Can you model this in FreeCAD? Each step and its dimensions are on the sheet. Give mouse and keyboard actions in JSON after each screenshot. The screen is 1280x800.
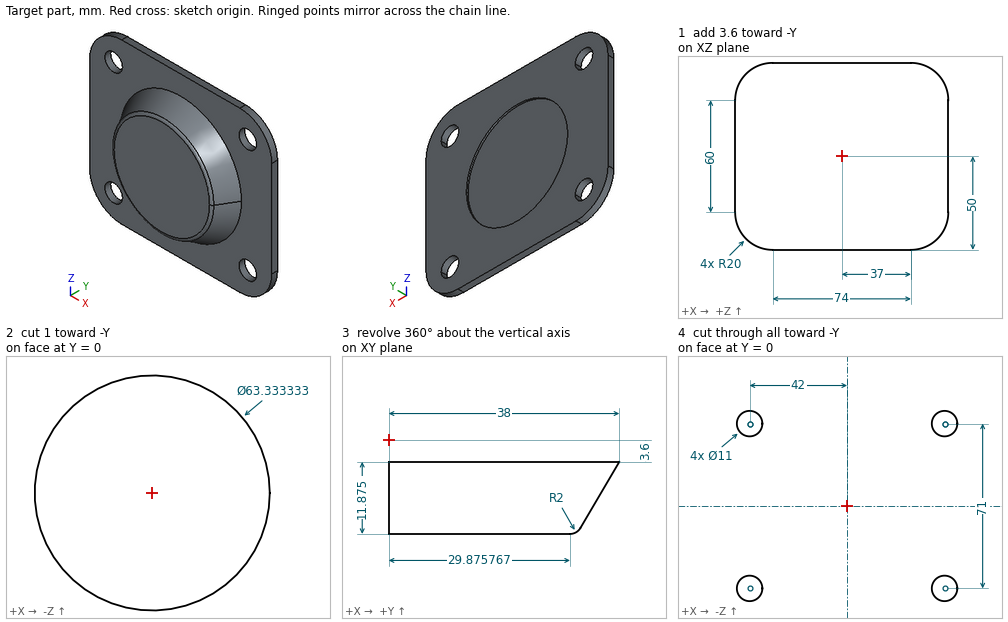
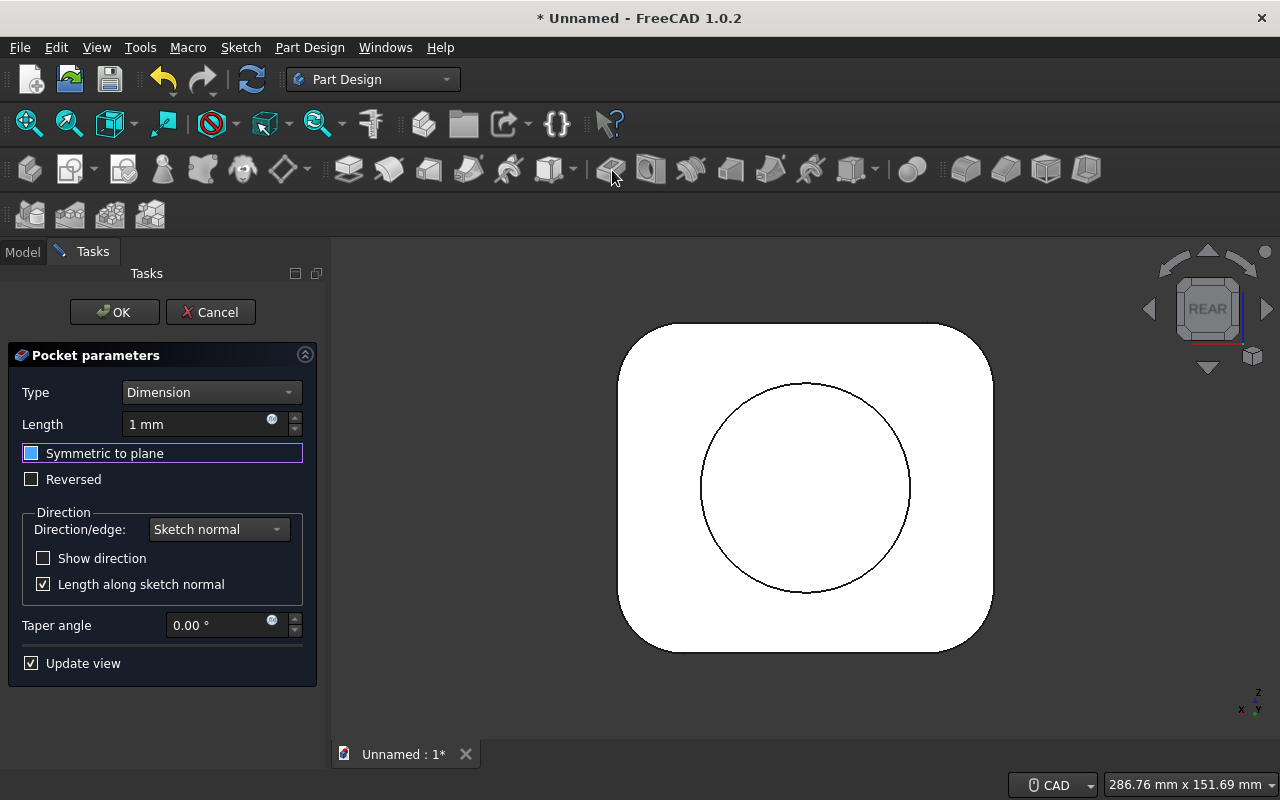
{"action": "left_click", "coordinate": [115, 312]}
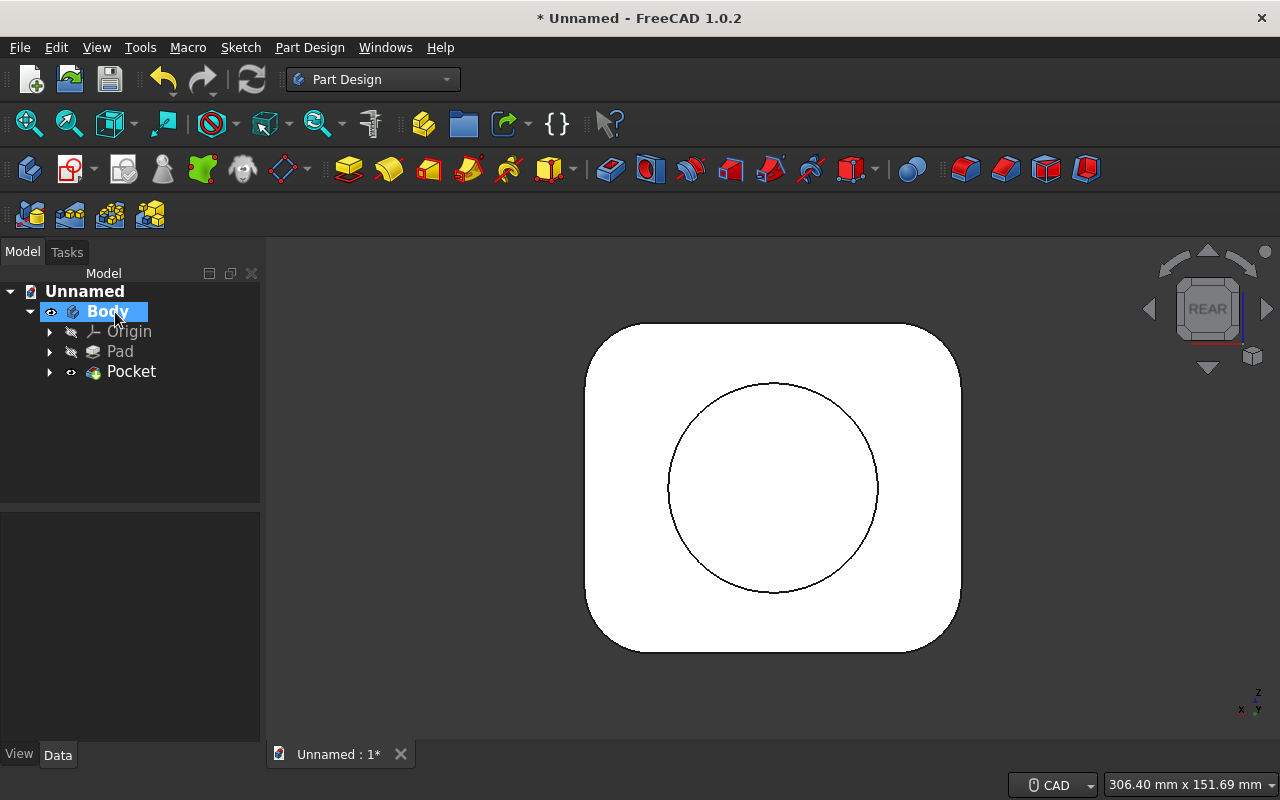
{"action": "left_click", "coordinate": [70, 170]}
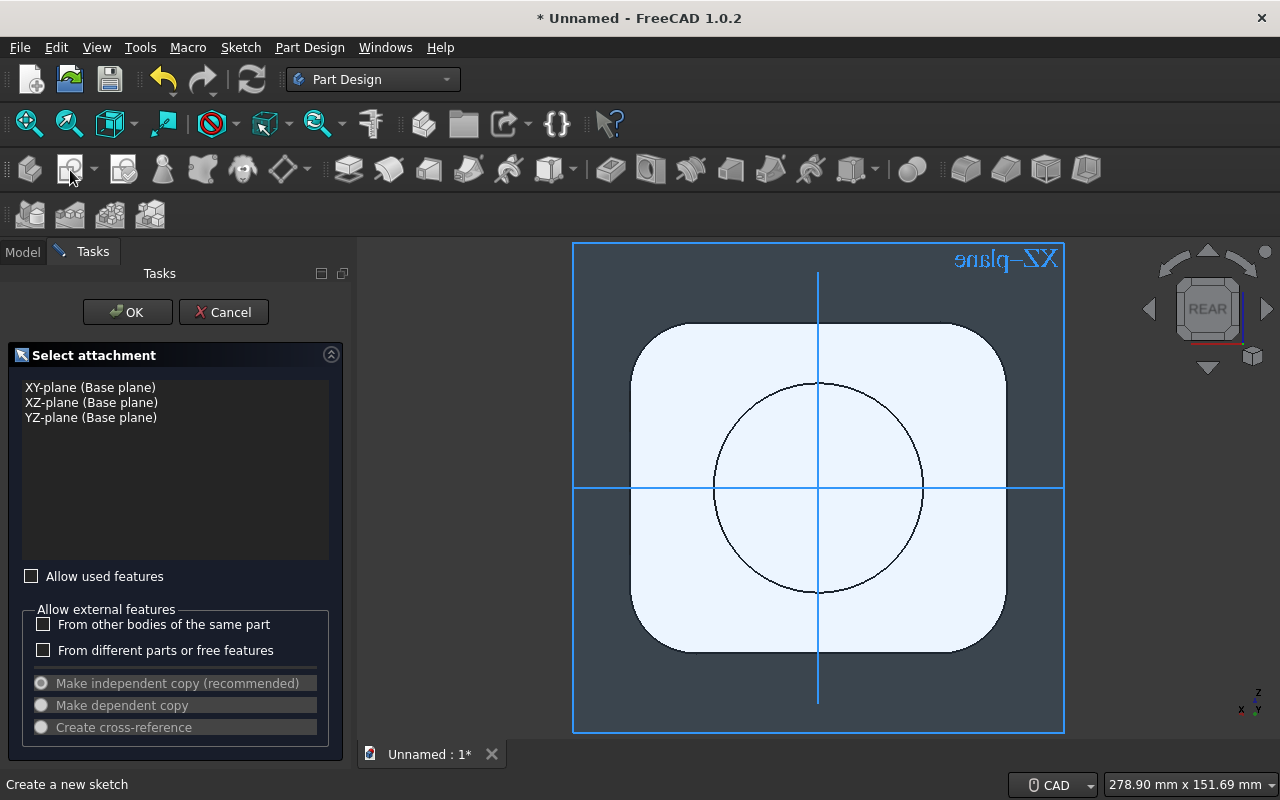
{"action": "left_click", "coordinate": [82, 388]}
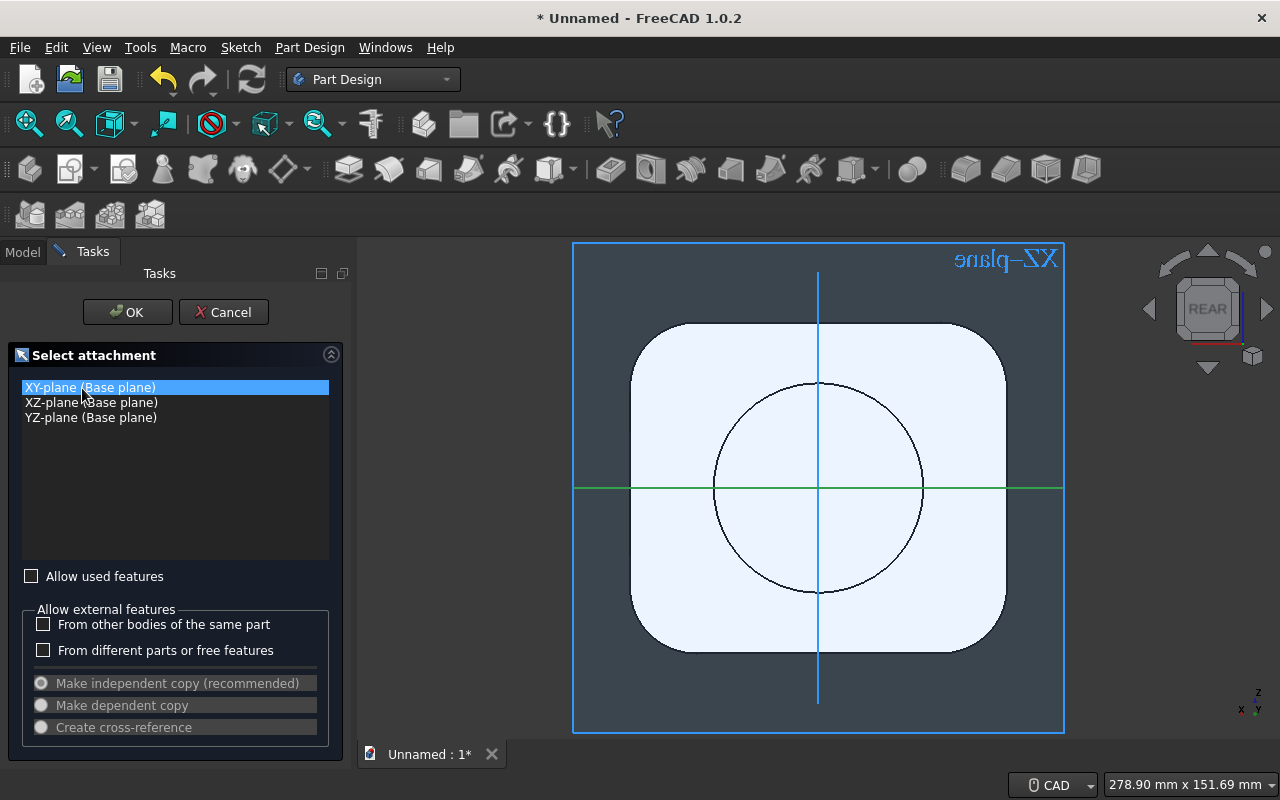
{"action": "left_click", "coordinate": [128, 312]}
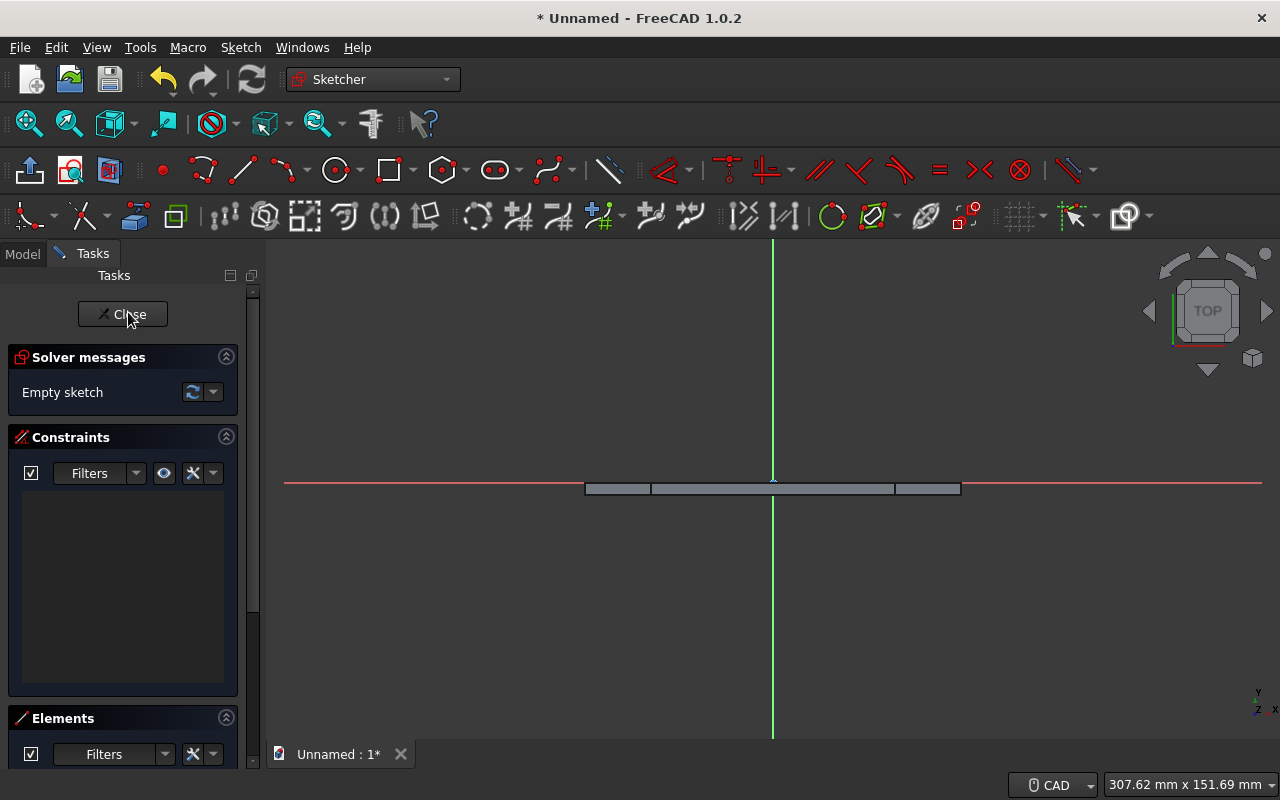
{"action": "left_click", "coordinate": [110, 170]}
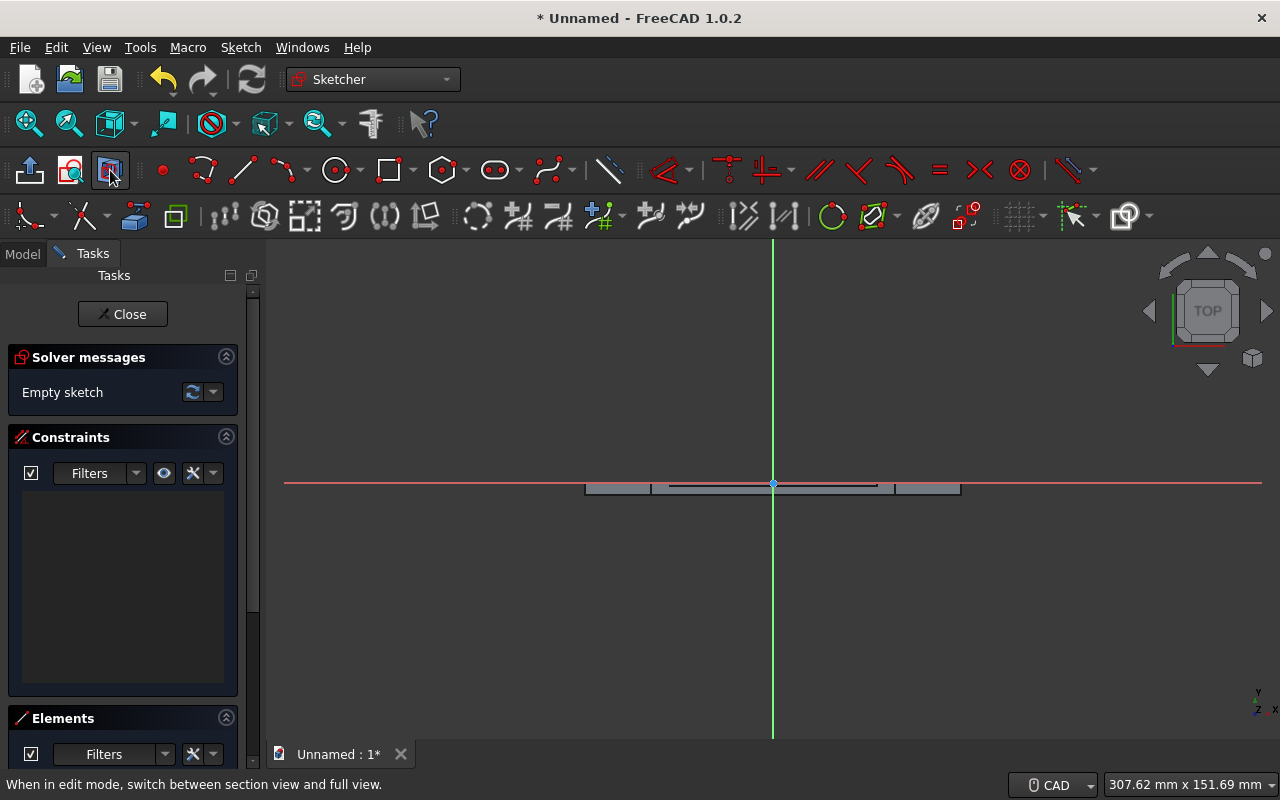
{"action": "scroll", "coordinate": [869, 514], "scroll_direction": "up", "scroll_amount": 8}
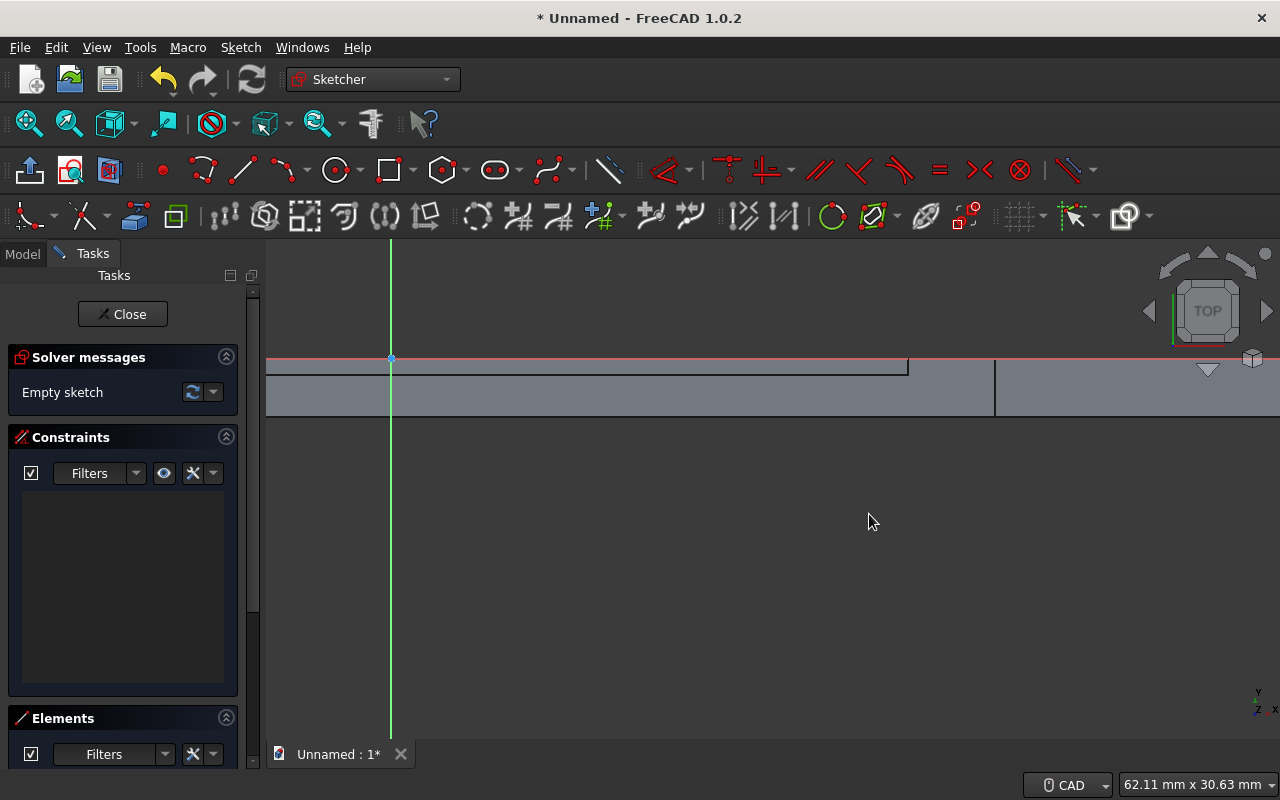
{"action": "left_click", "coordinate": [204, 170]}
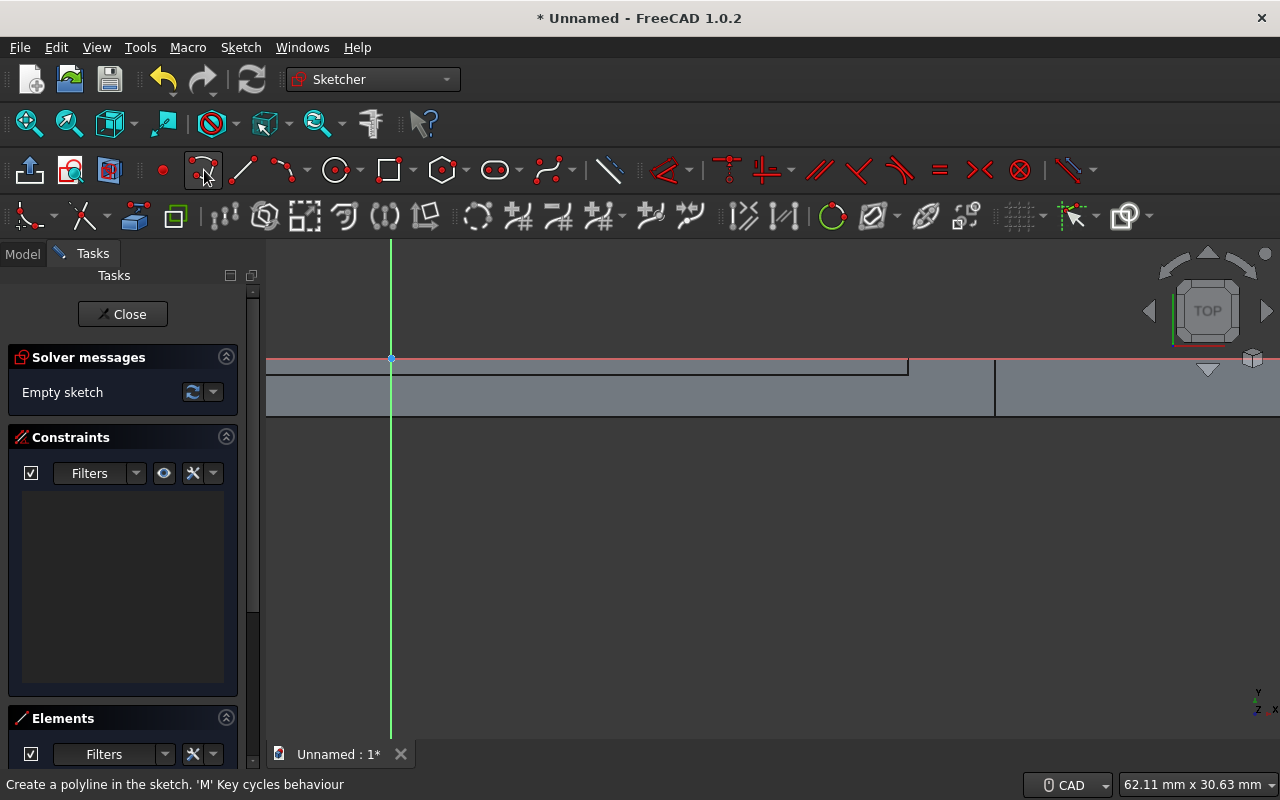
{"action": "left_click", "coordinate": [907, 595]}
{"action": "left_click", "coordinate": [1012, 417]}
{"action": "left_click", "coordinate": [391, 417]}
{"action": "left_click", "coordinate": [400, 611]}
{"action": "left_click", "coordinate": [879, 611]}
{"action": "right_click", "coordinate": [879, 611]}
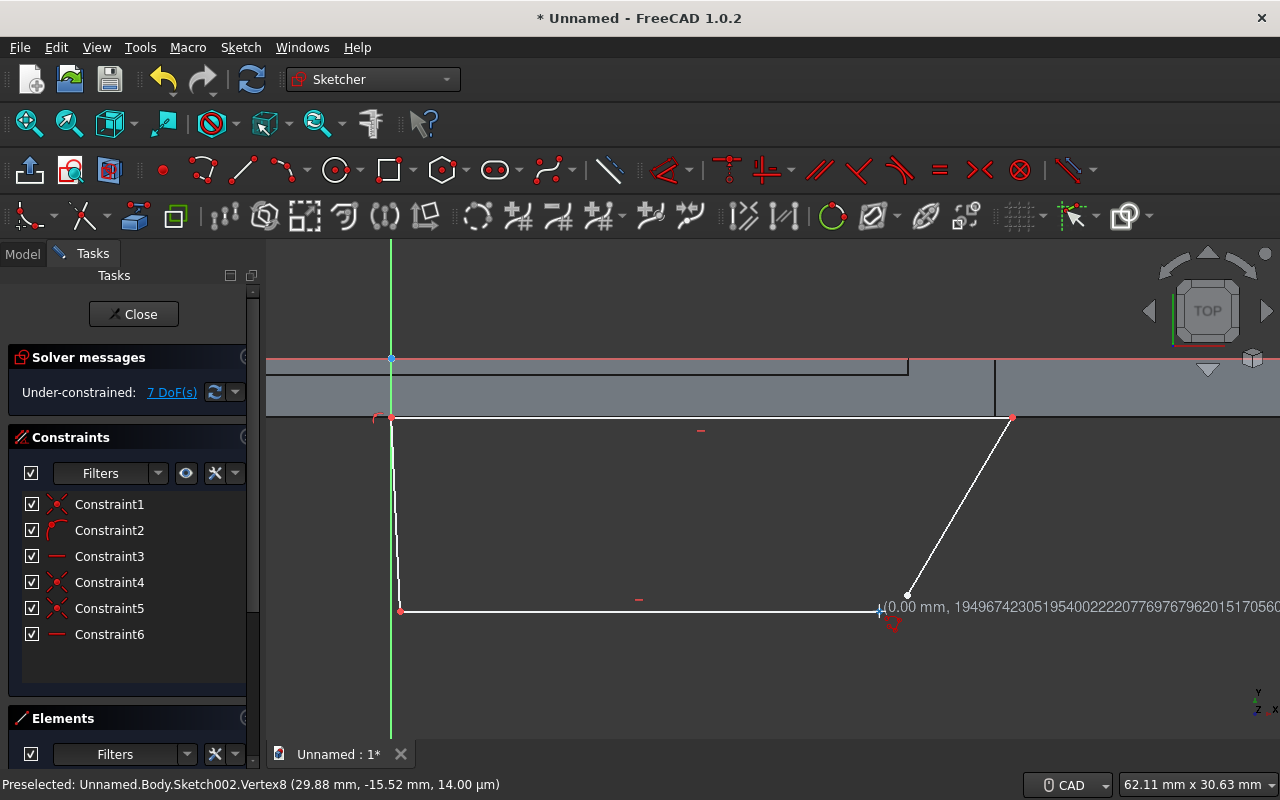
{"action": "left_click", "coordinate": [284, 170]}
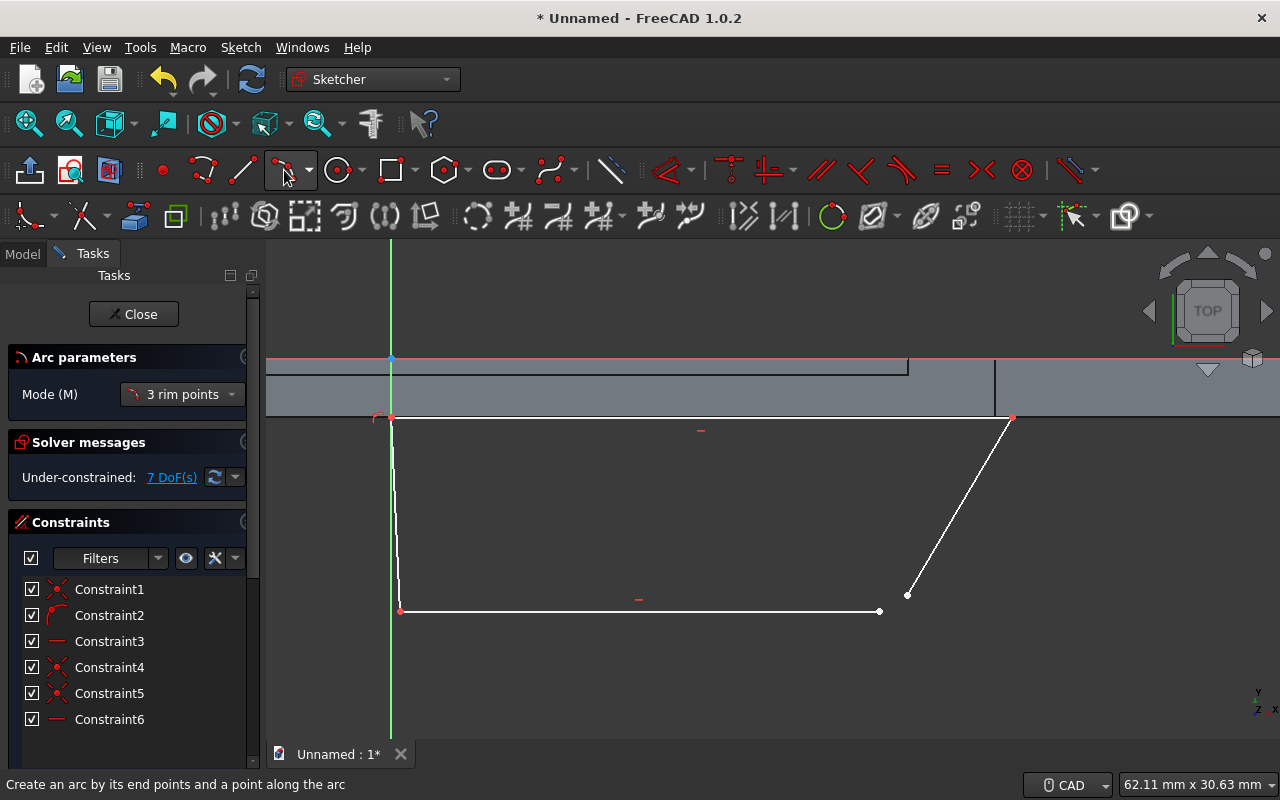
{"action": "left_click", "coordinate": [879, 612]}
{"action": "left_click", "coordinate": [907, 596]}